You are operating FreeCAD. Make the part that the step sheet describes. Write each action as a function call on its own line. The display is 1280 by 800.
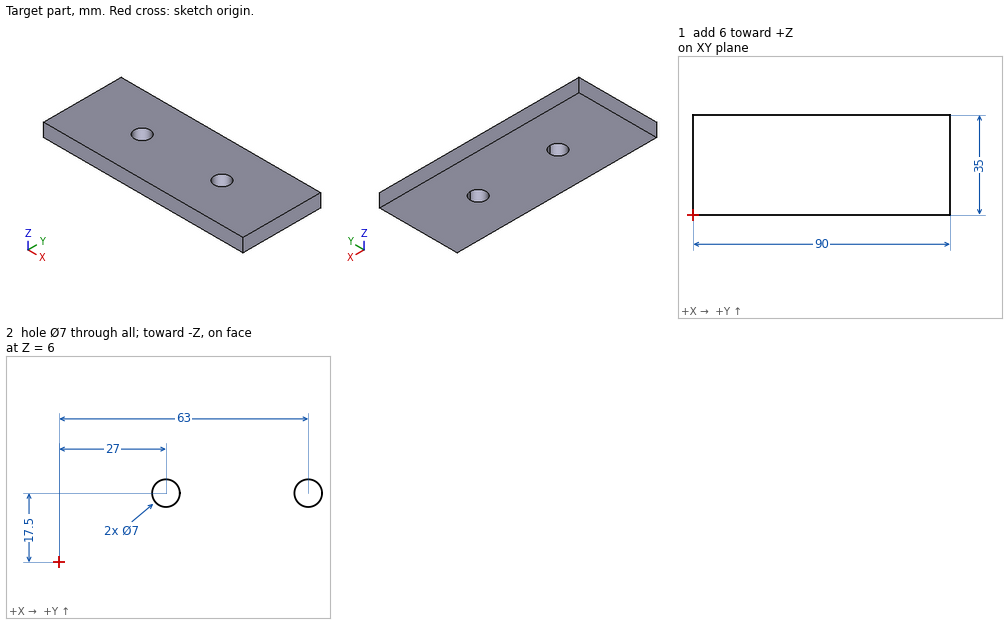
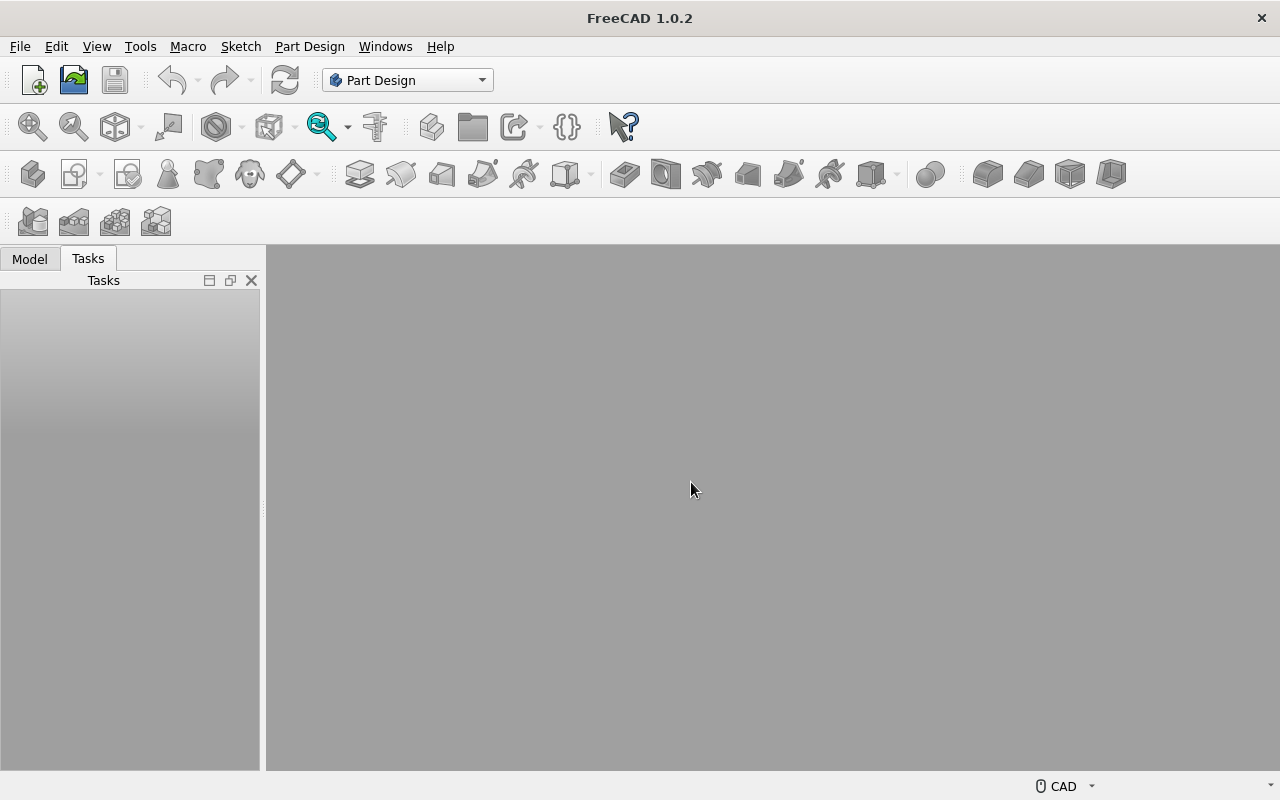
click(33, 80)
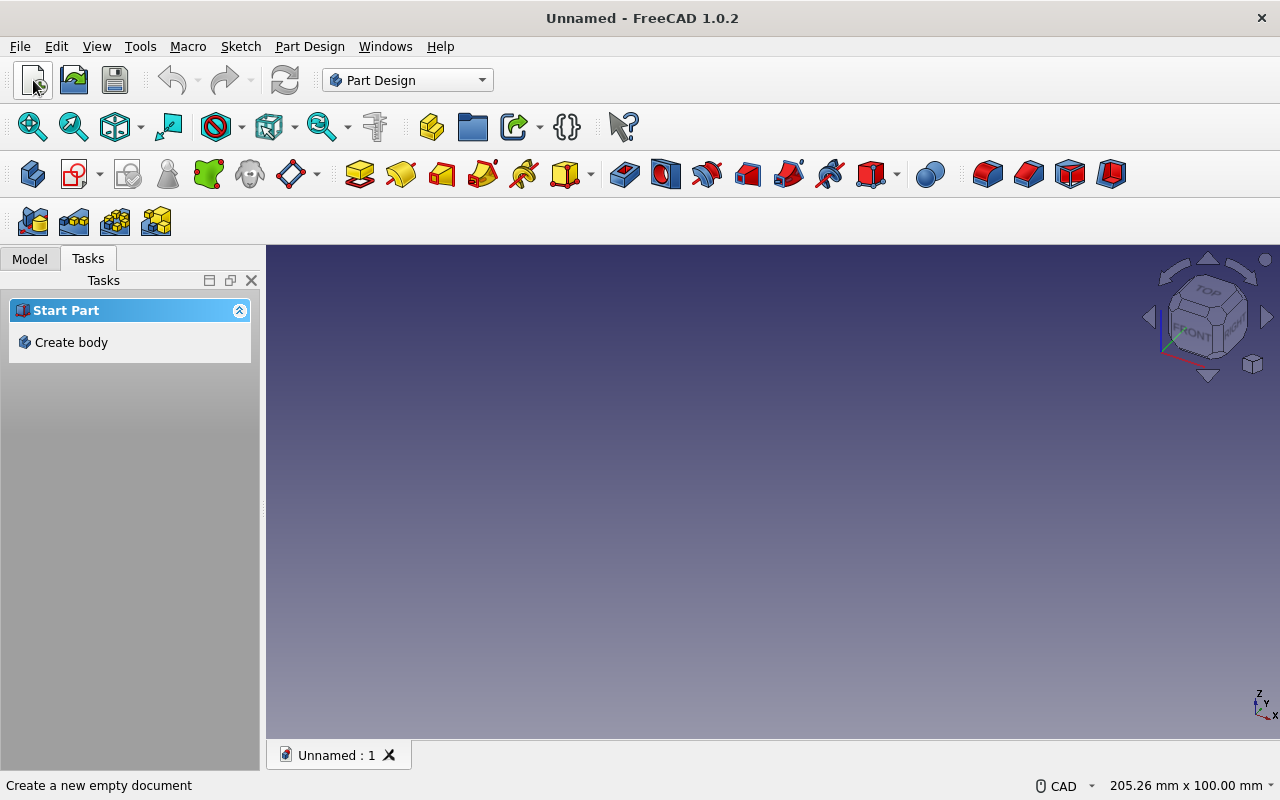
click(74, 174)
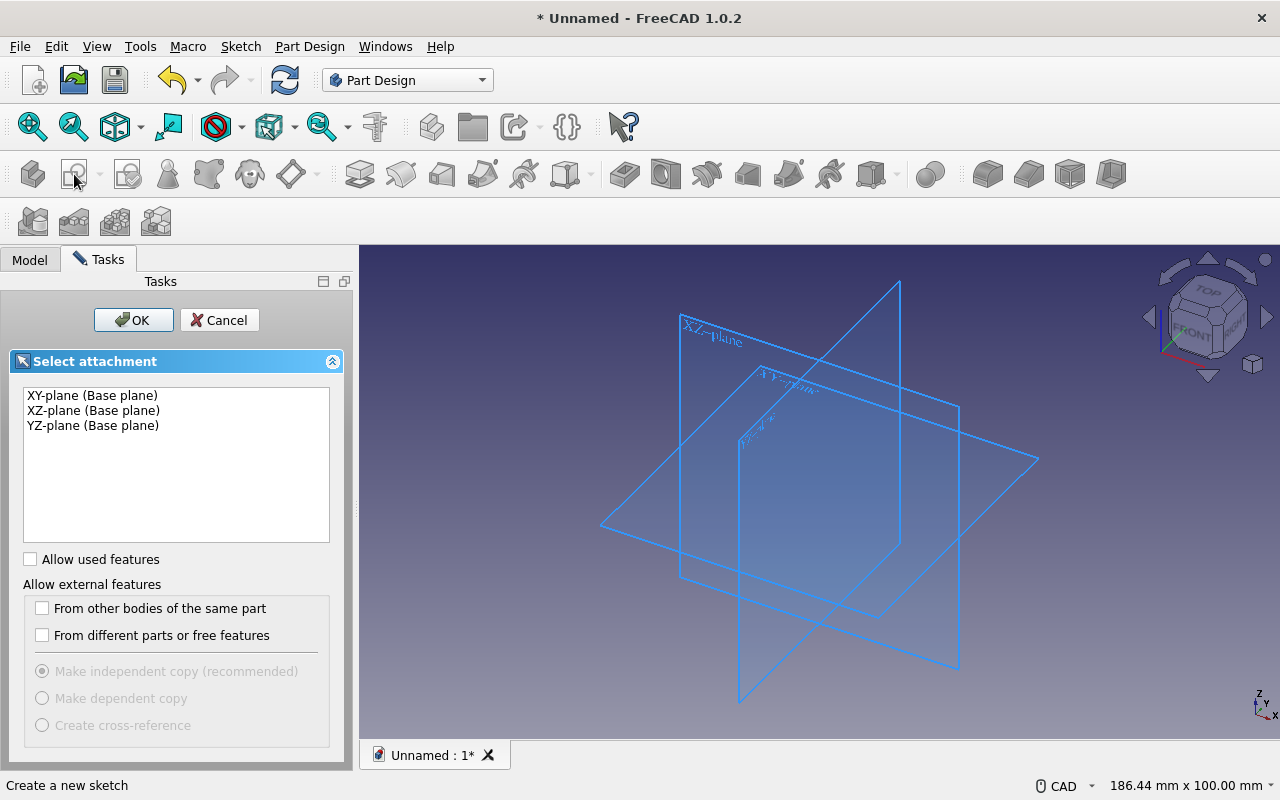
click(84, 396)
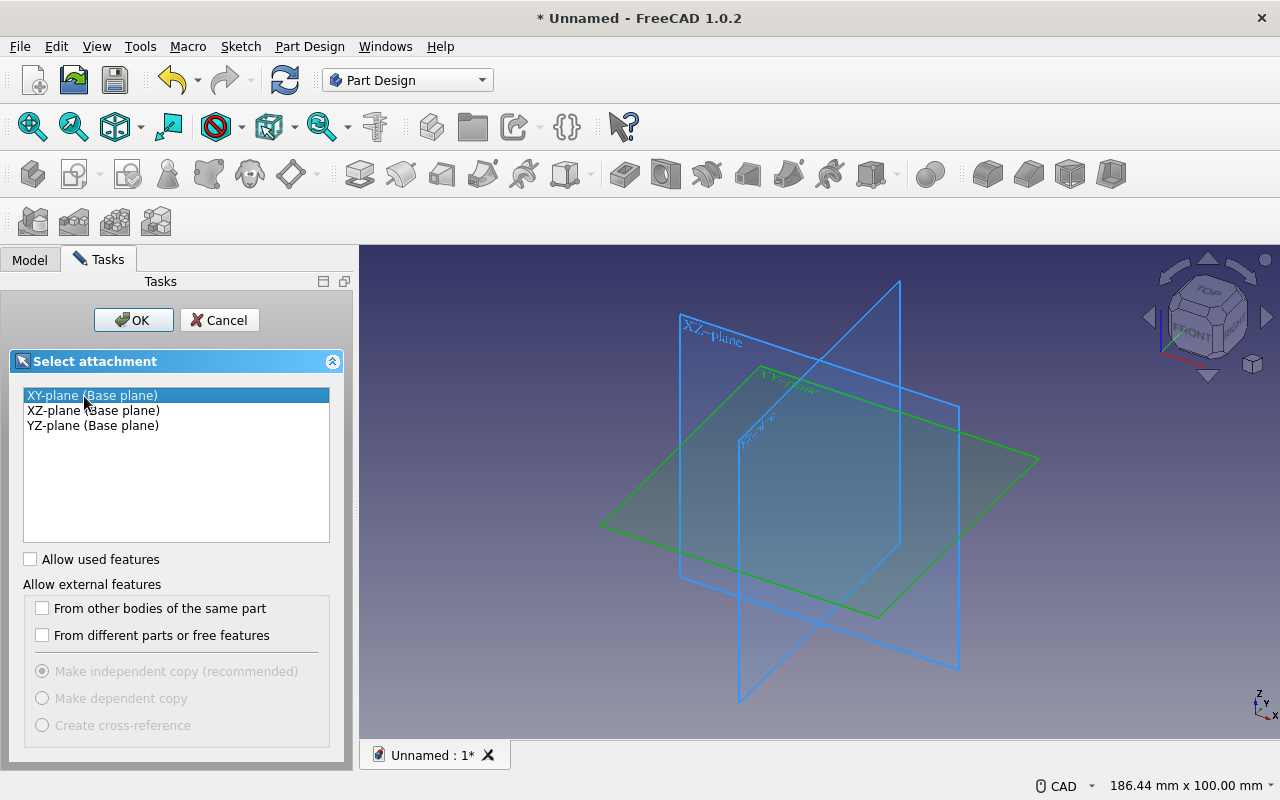
click(134, 320)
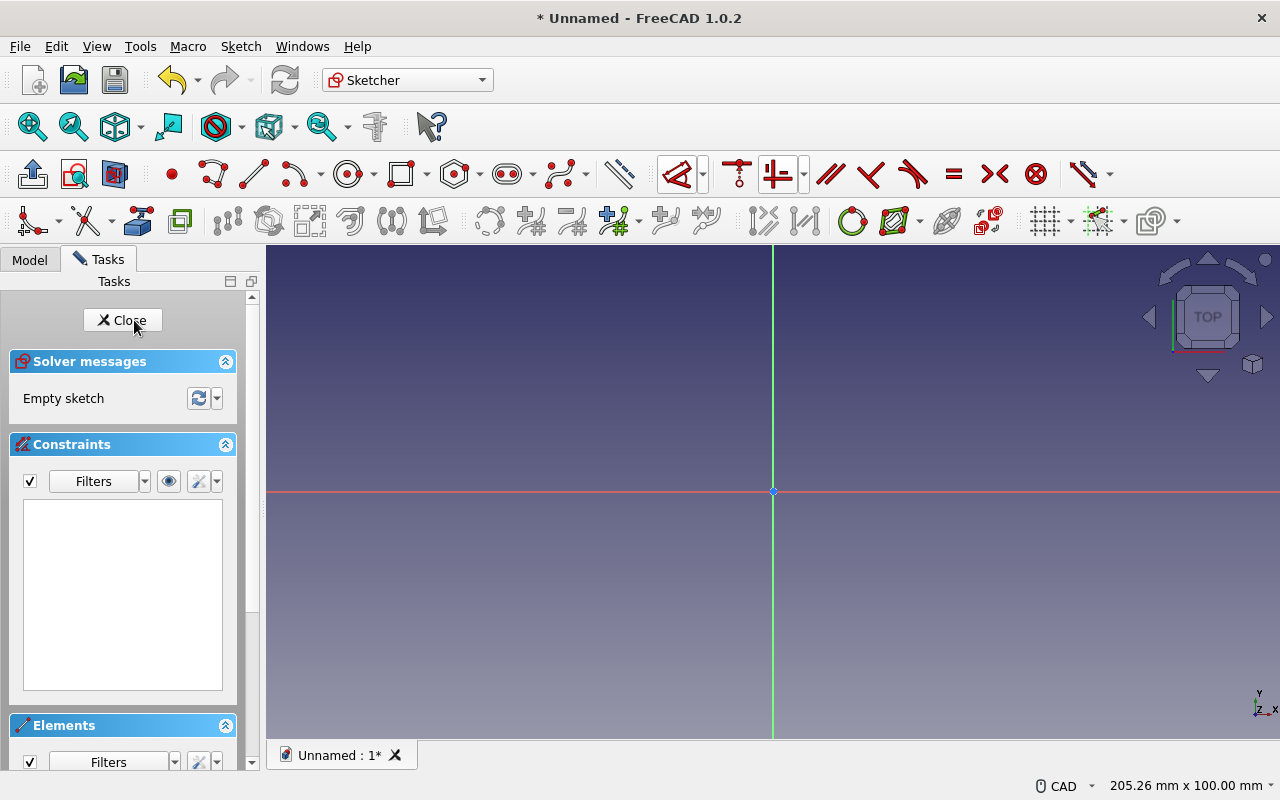
scroll(294, 711, down, 1)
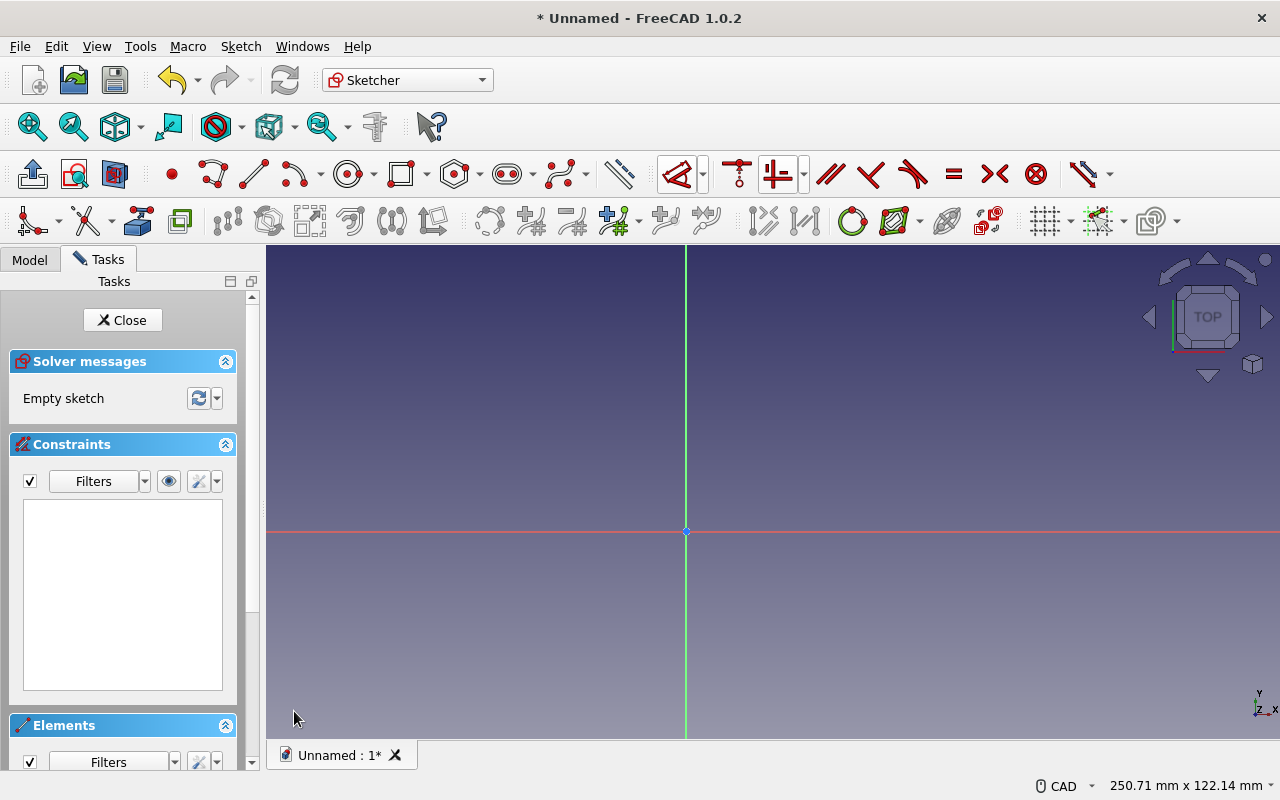
scroll(1115, 398, up, 2)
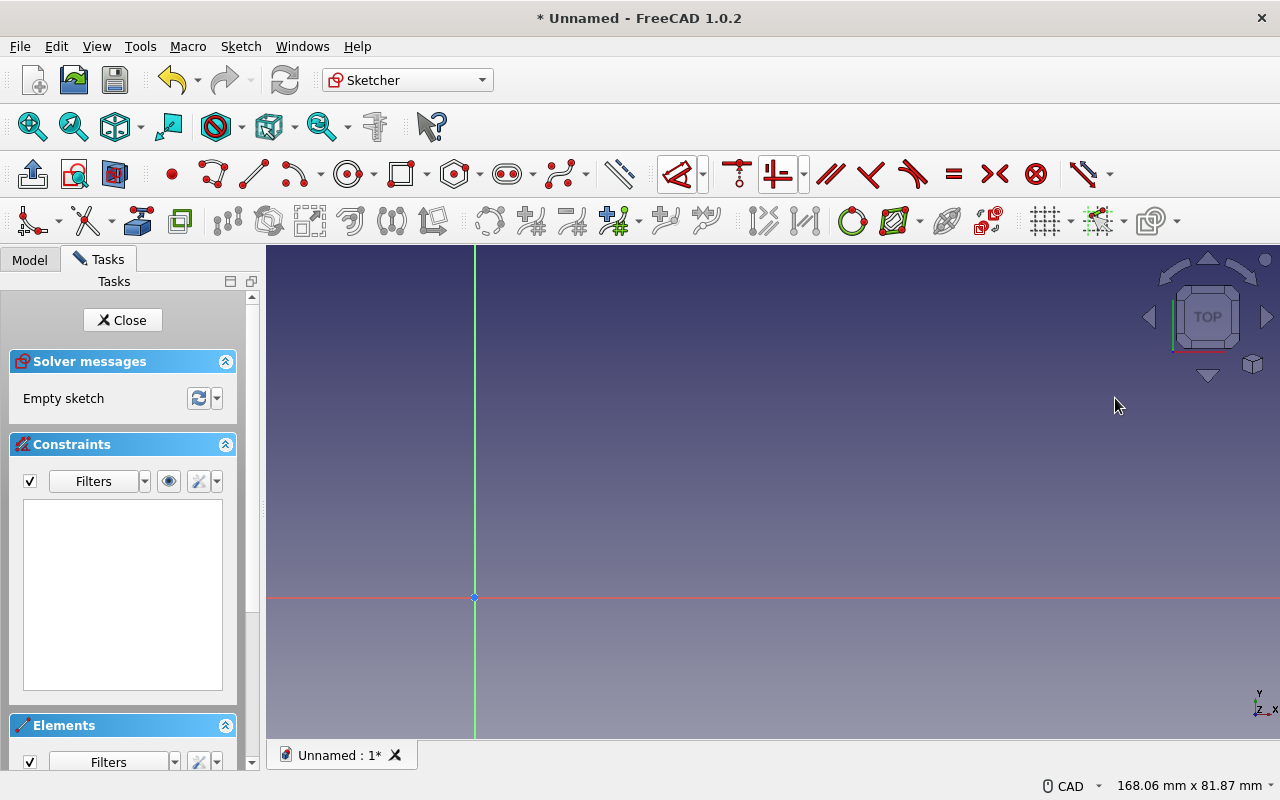
click(400, 174)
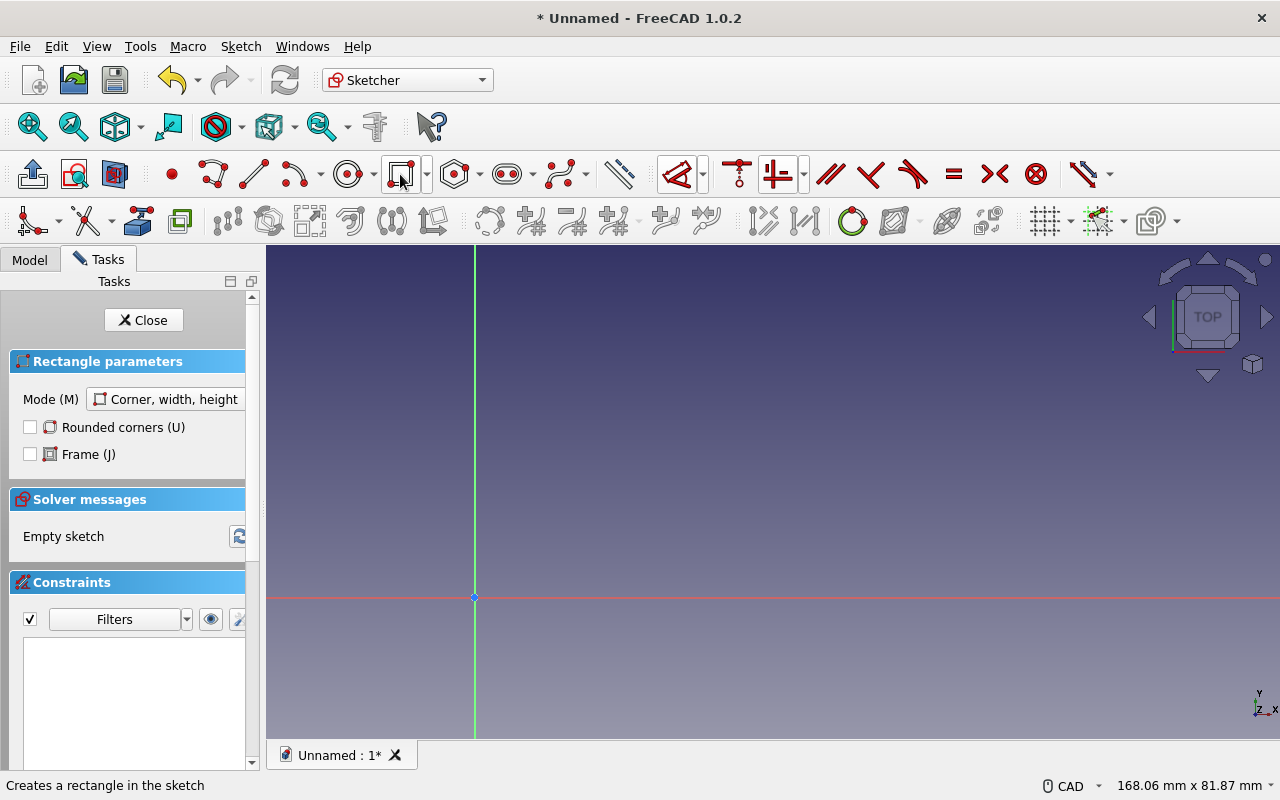
click(475, 598)
click(1018, 386)
key(Escape)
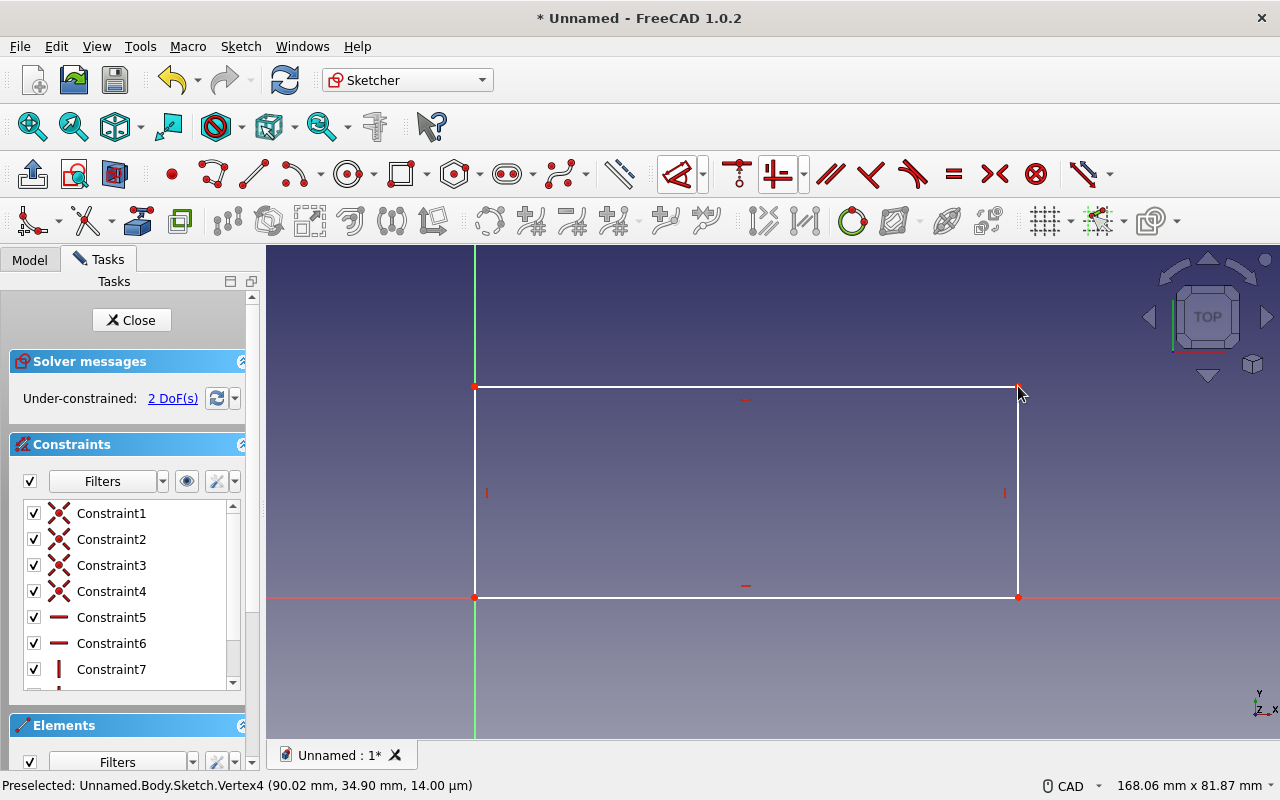
click(638, 598)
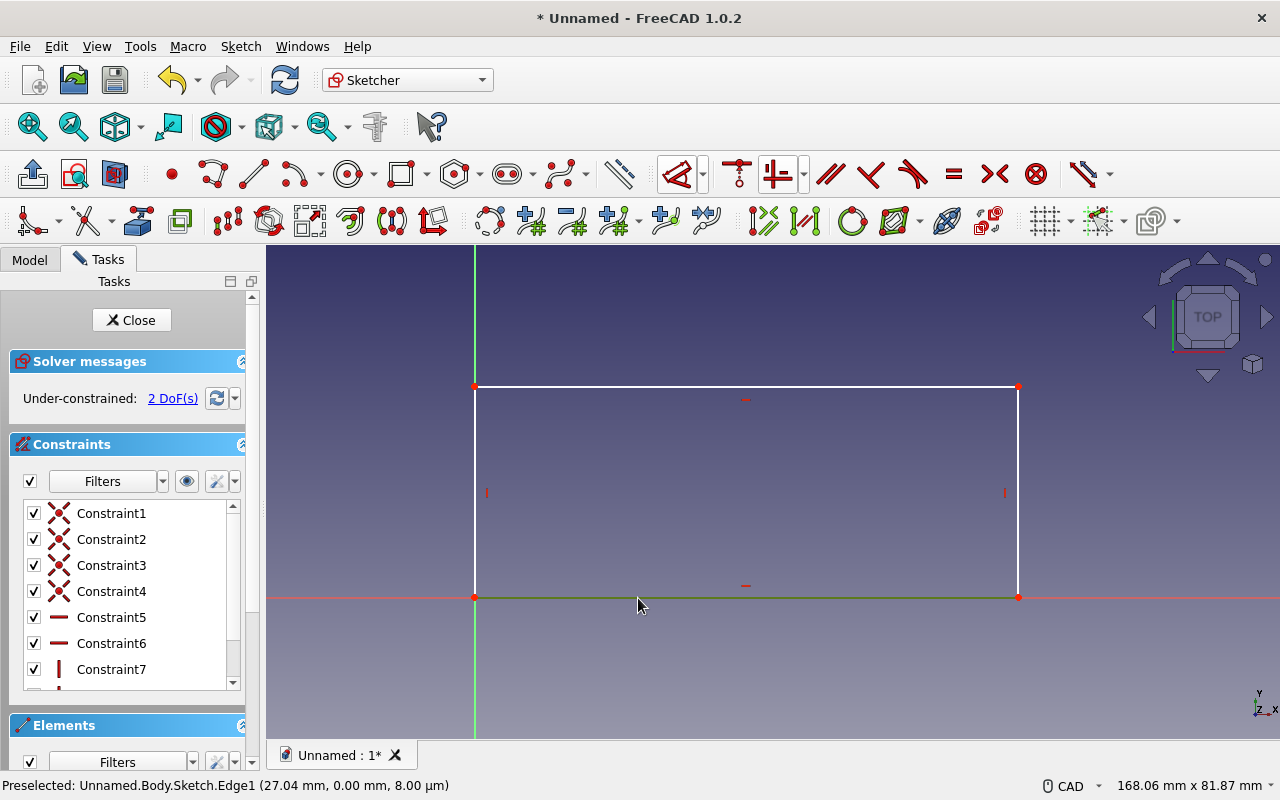
key(l)